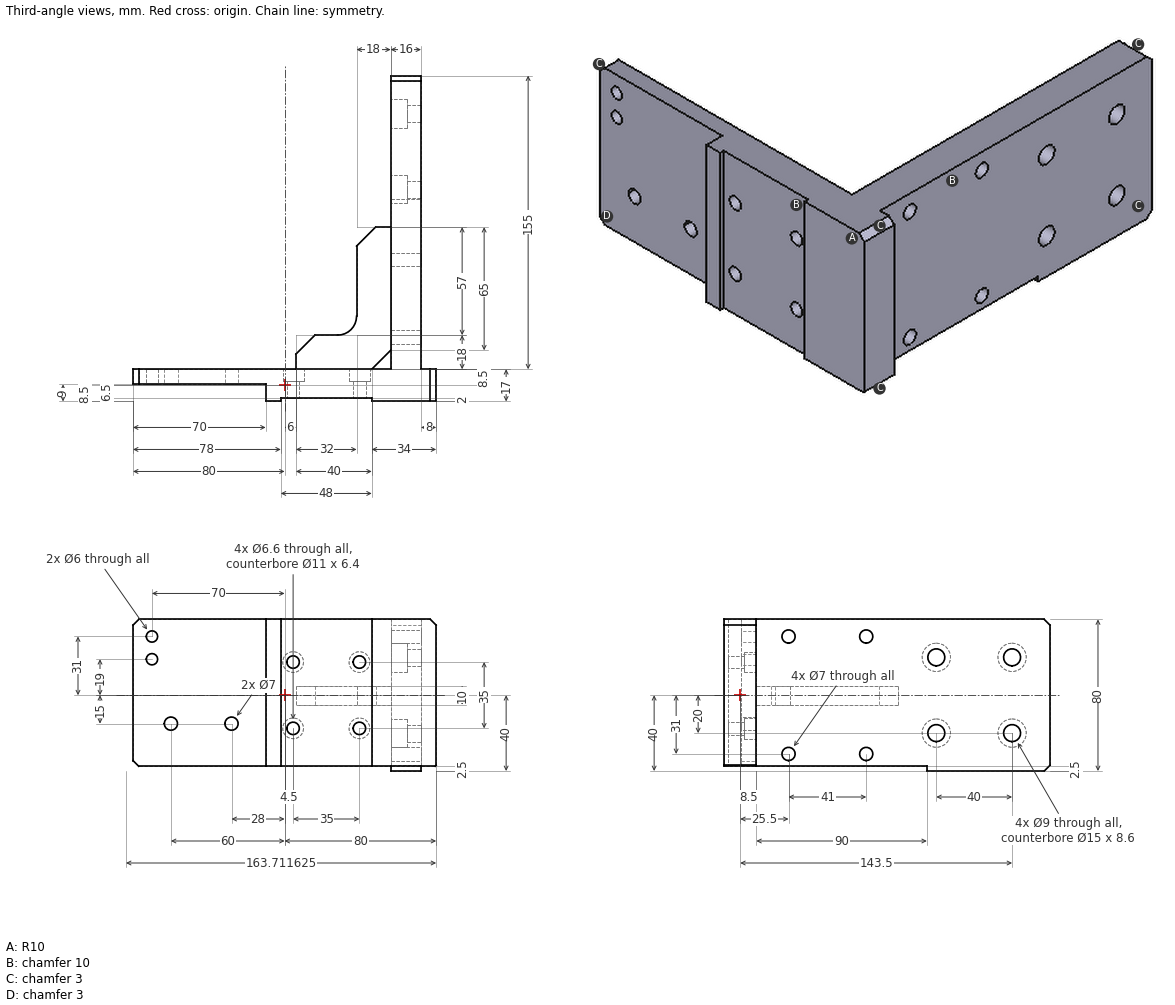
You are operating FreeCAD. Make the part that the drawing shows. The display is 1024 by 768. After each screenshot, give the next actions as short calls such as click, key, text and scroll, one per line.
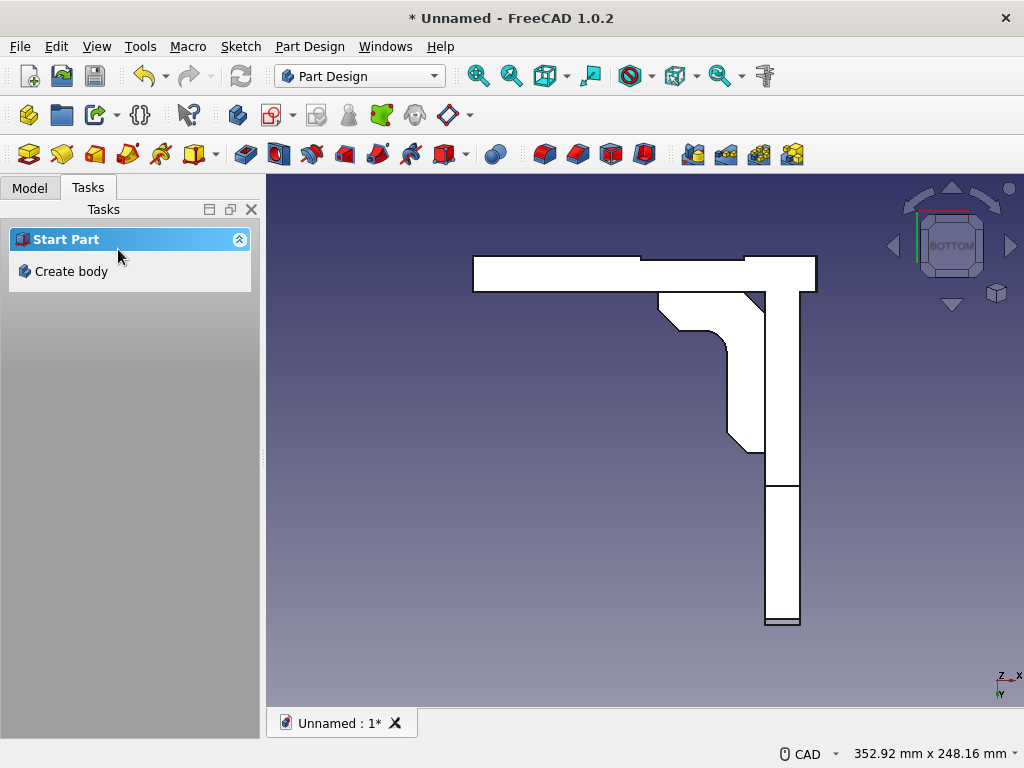
click(791, 271)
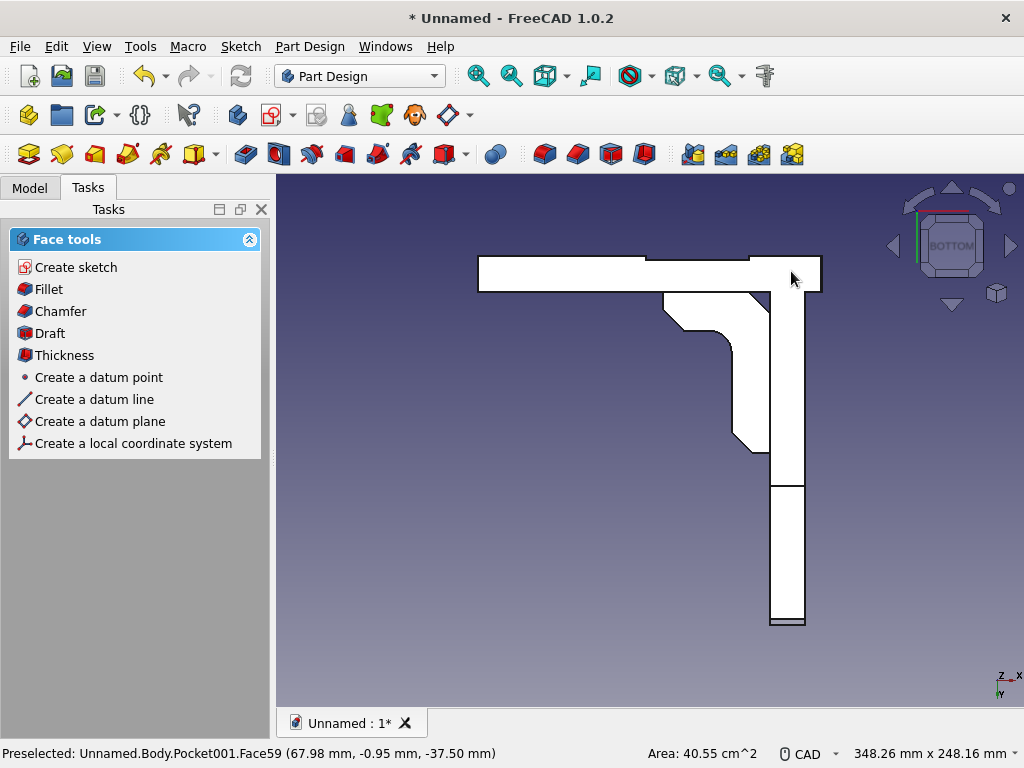
click(270, 116)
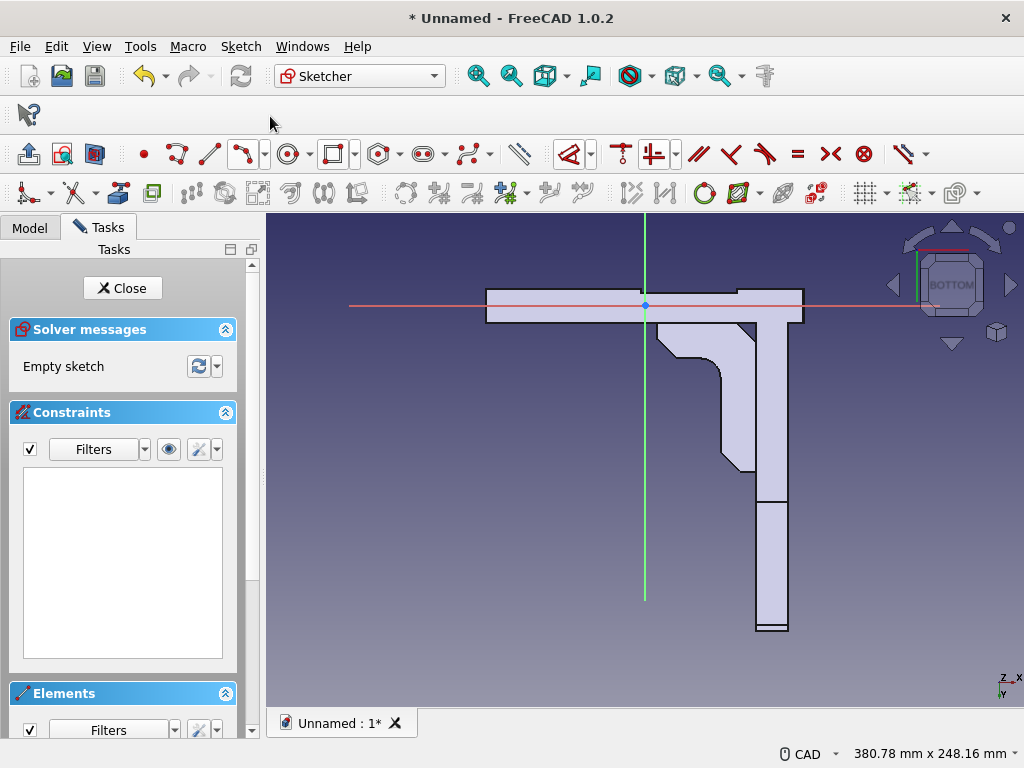
scroll(559, 241, up, 5)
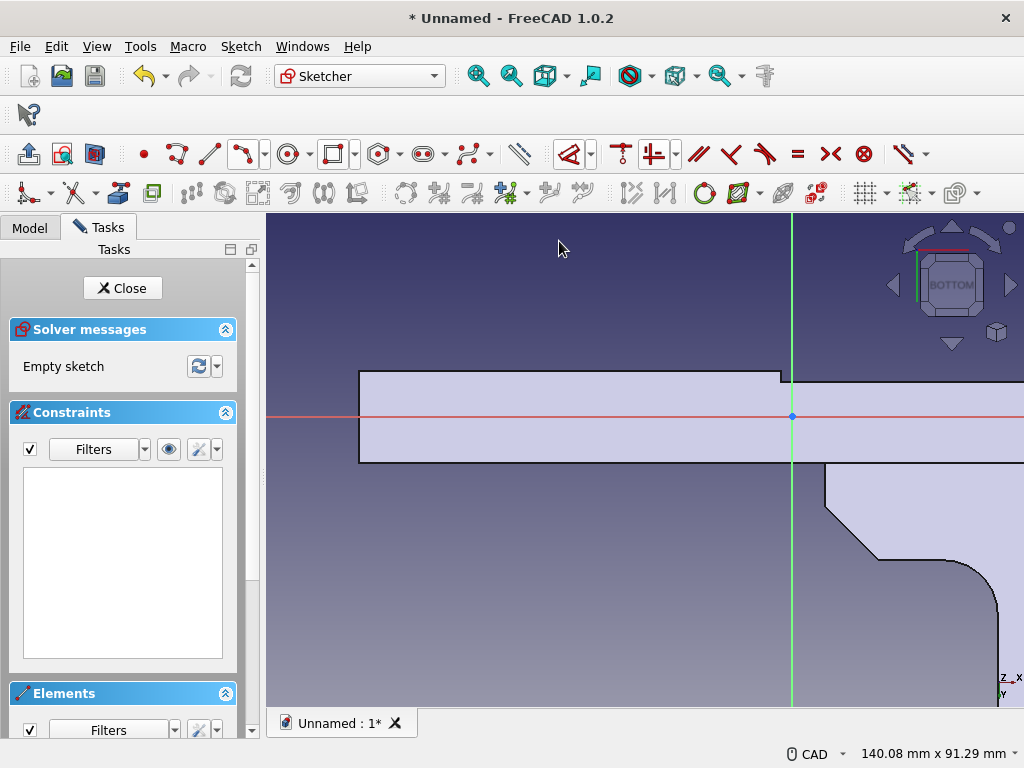
click(332, 154)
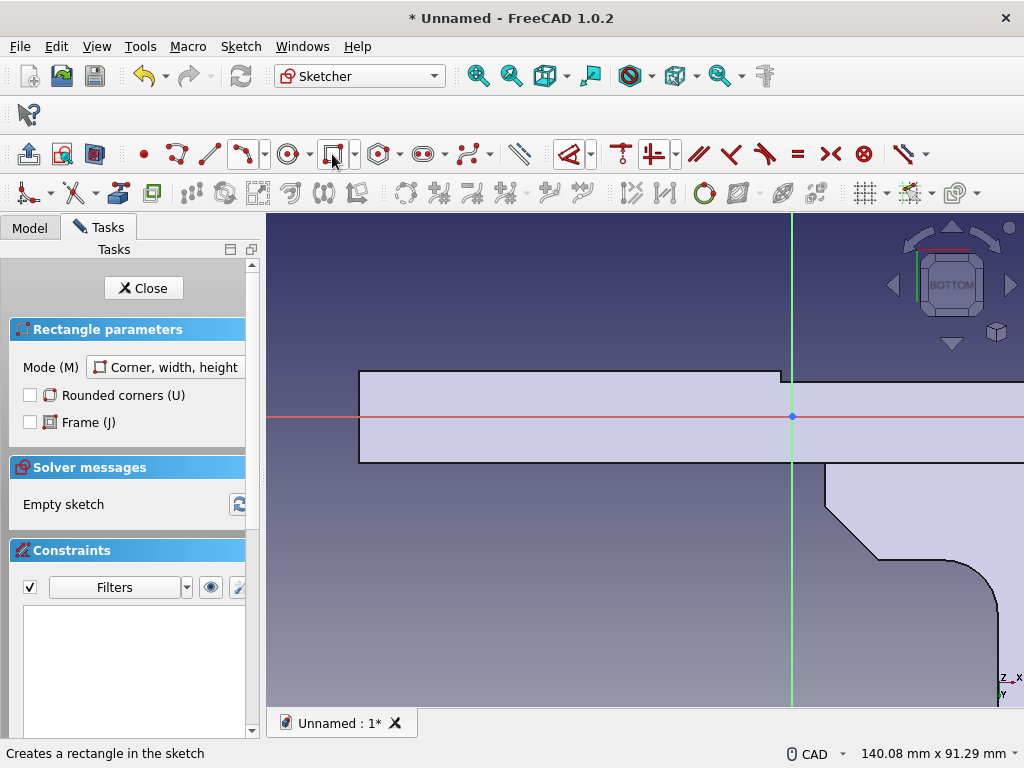
click(359, 371)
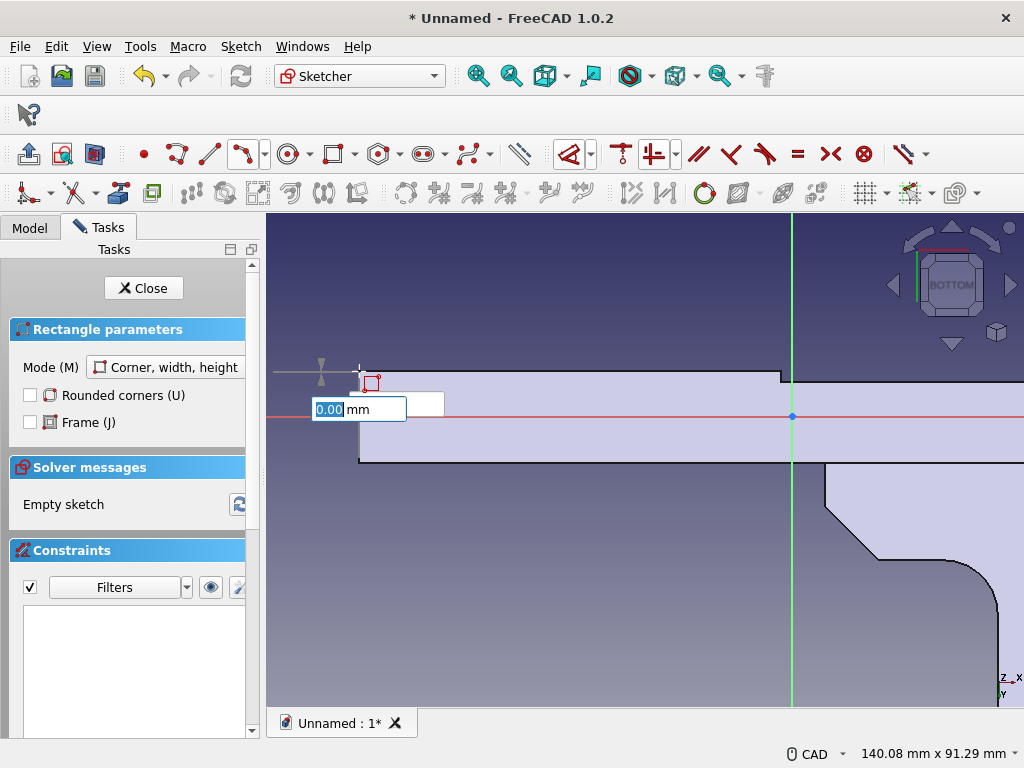
scroll(738, 420, up, 9)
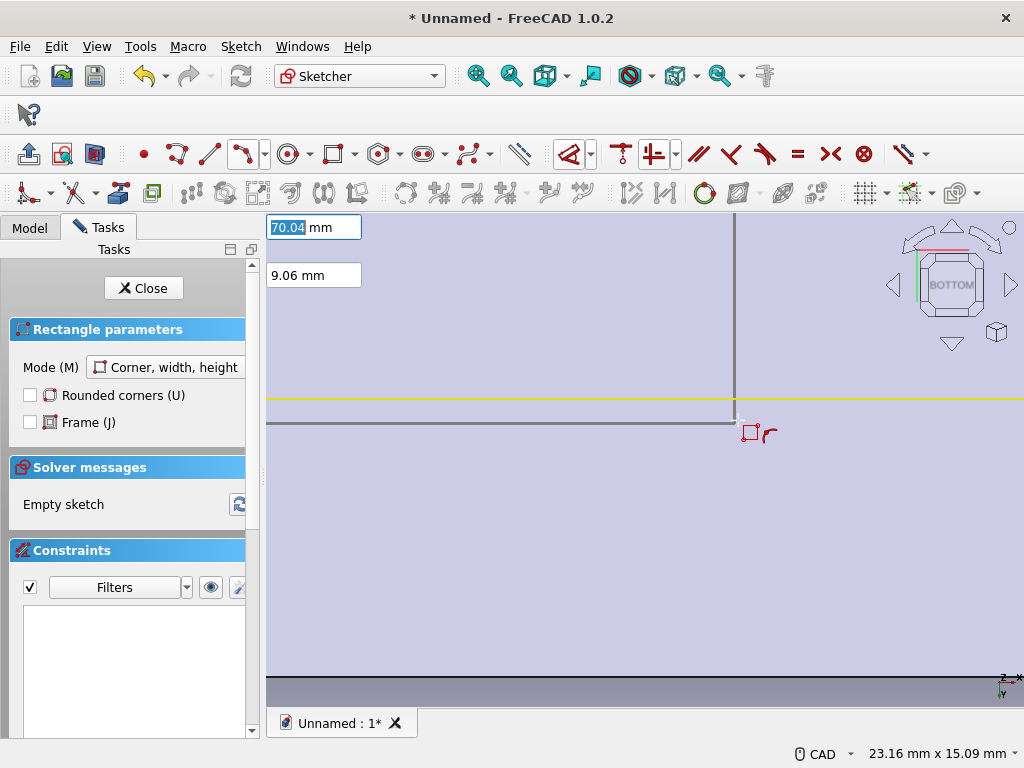
click(735, 415)
key(Escape)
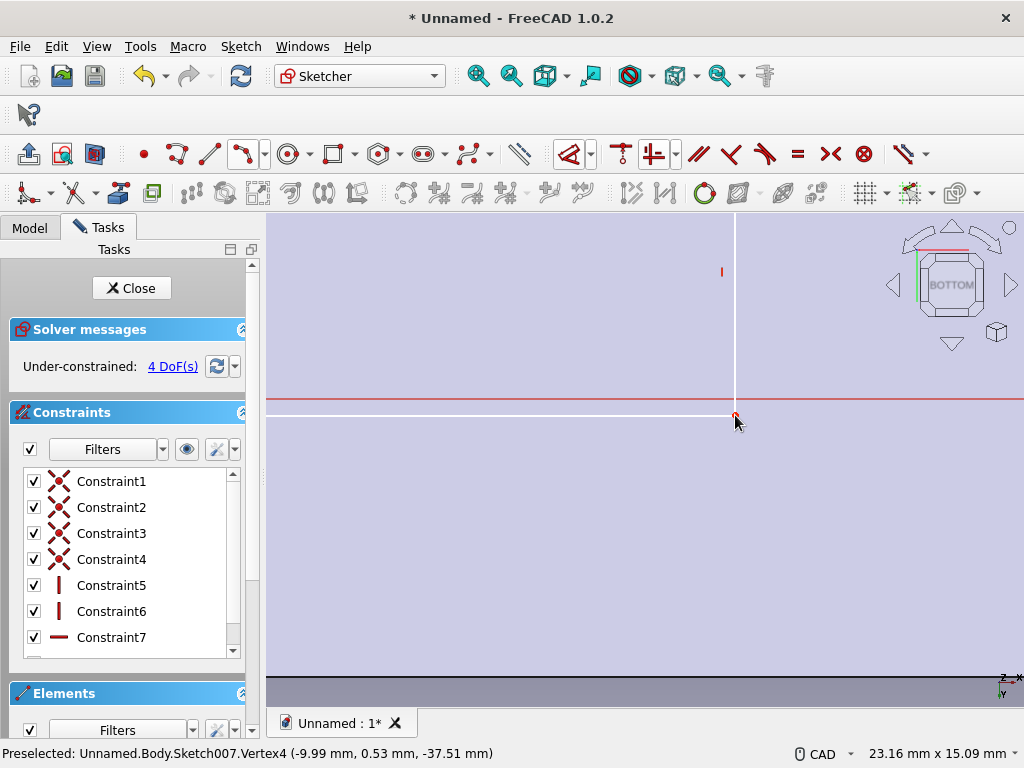
scroll(740, 498, down, 9)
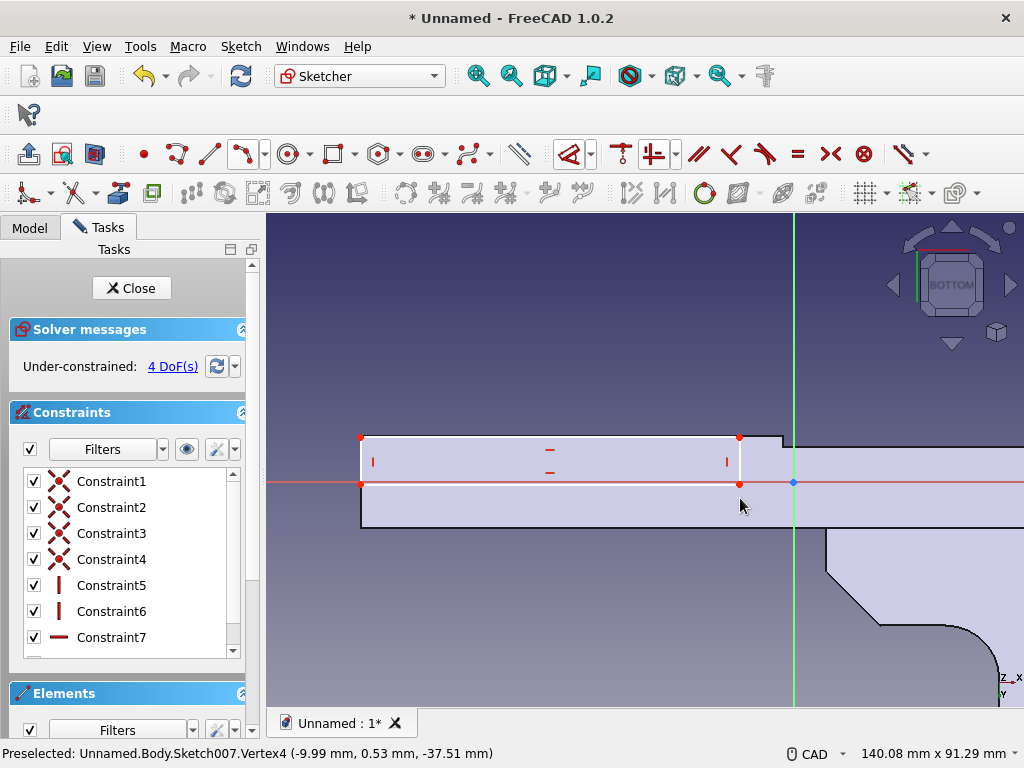
click(361, 452)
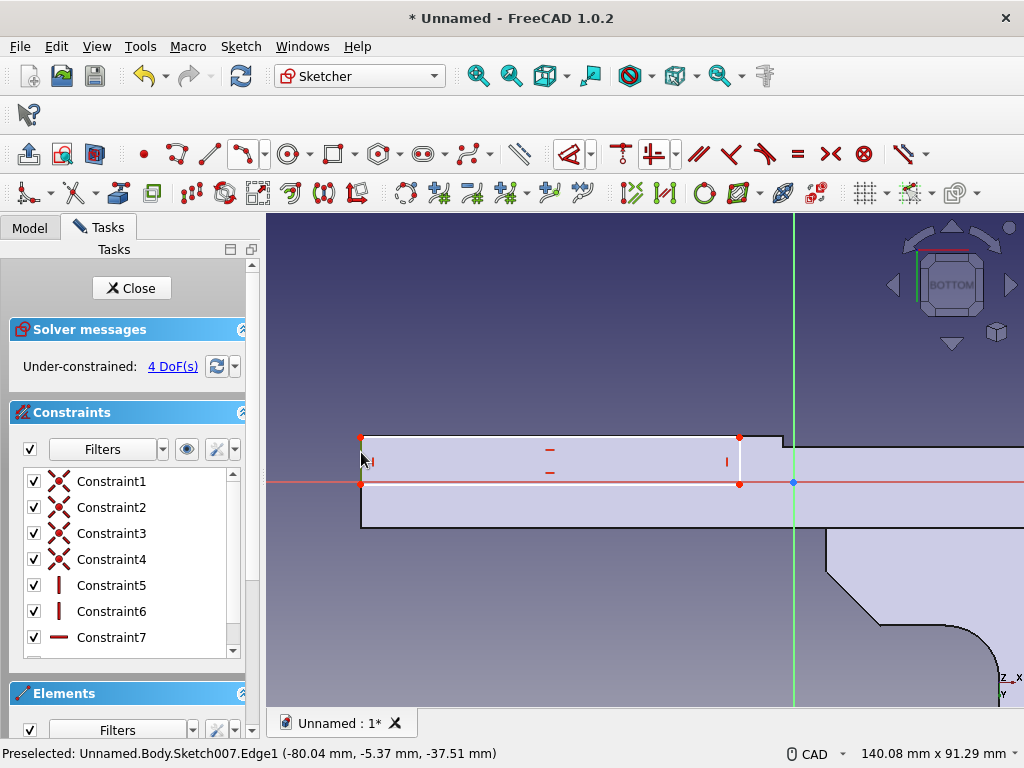
key(i)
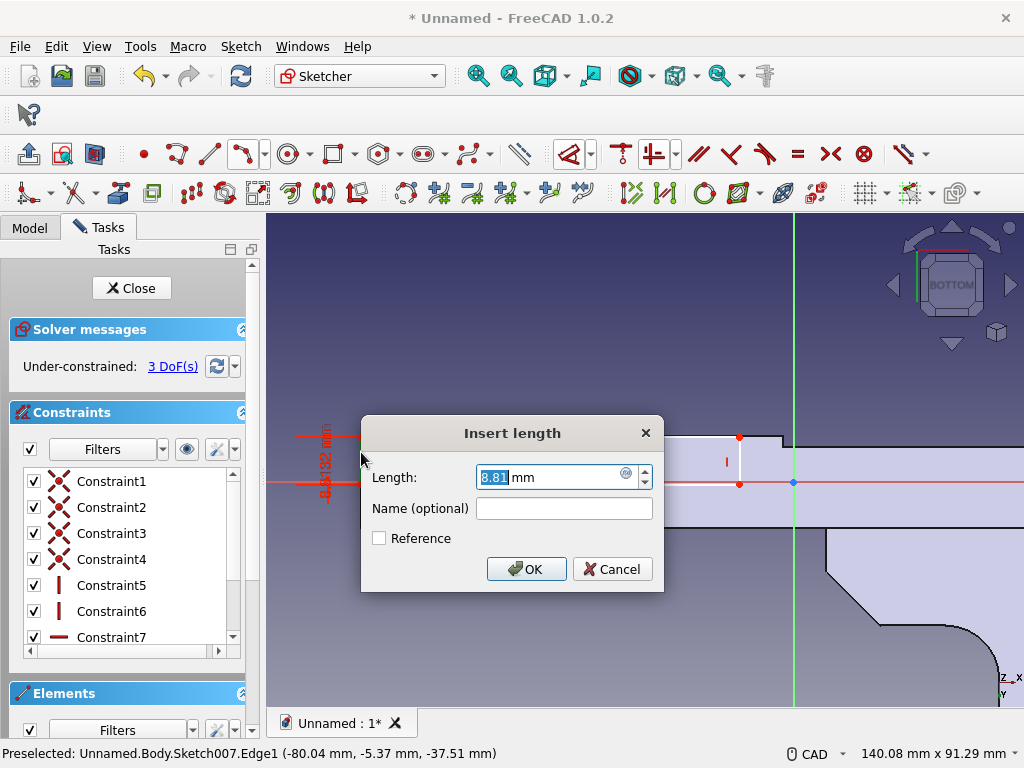
text(9)
key(Return)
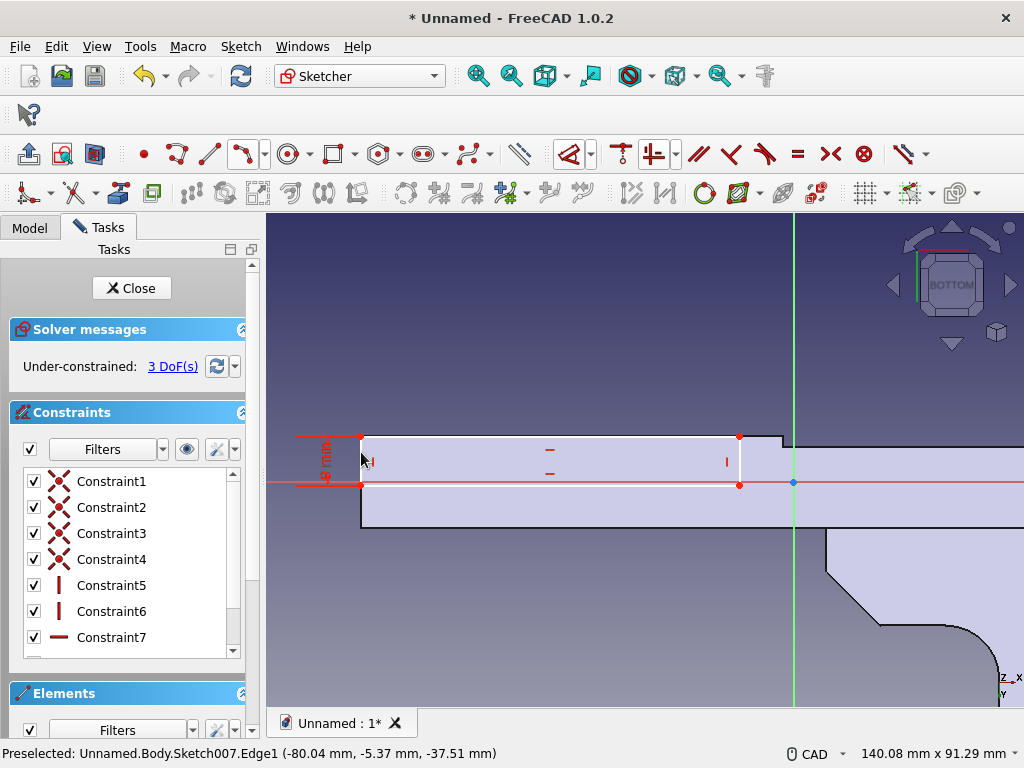
click(474, 486)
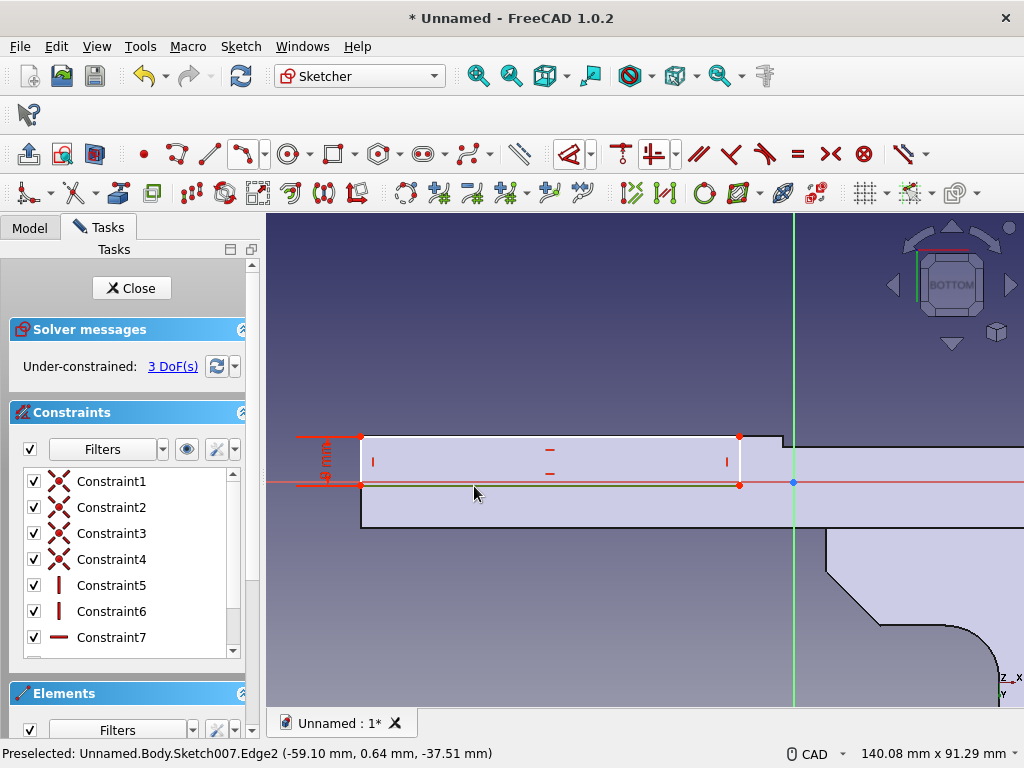
key(l)